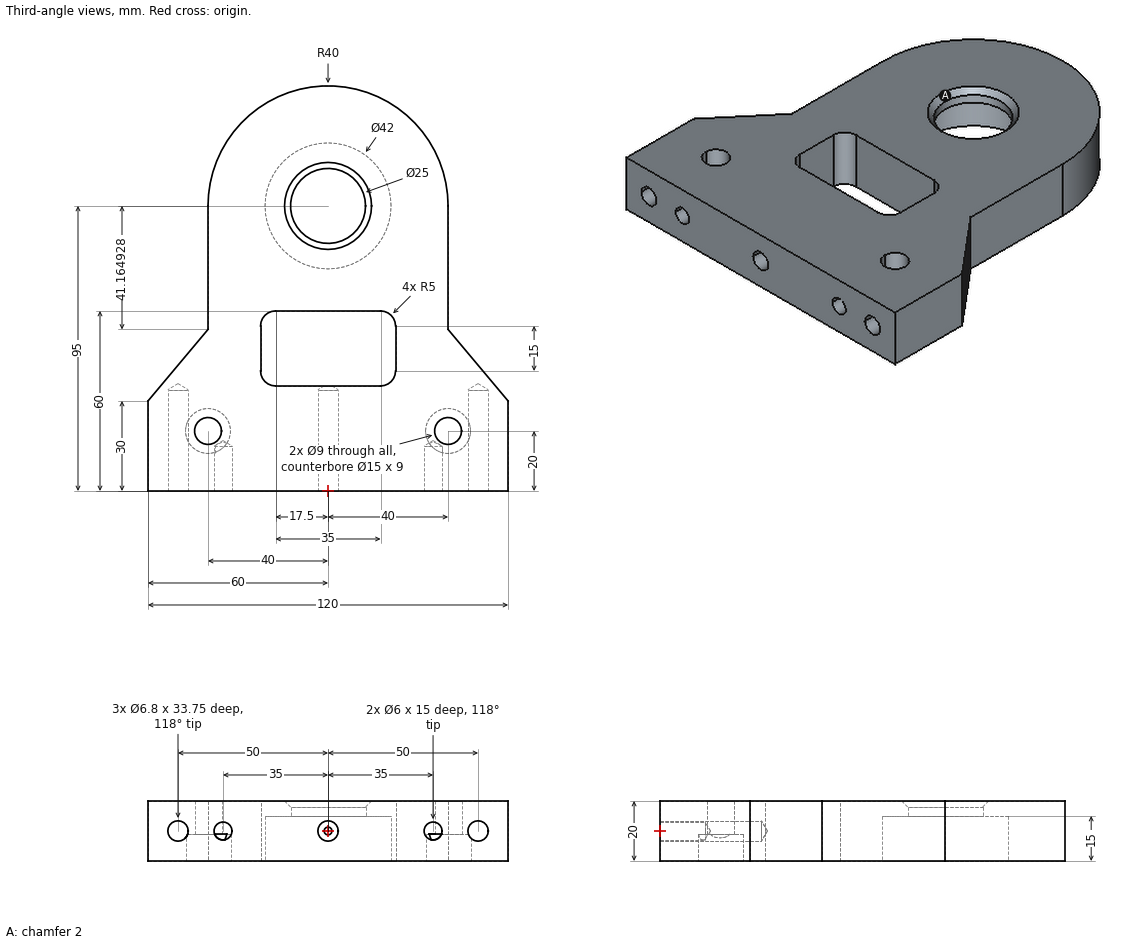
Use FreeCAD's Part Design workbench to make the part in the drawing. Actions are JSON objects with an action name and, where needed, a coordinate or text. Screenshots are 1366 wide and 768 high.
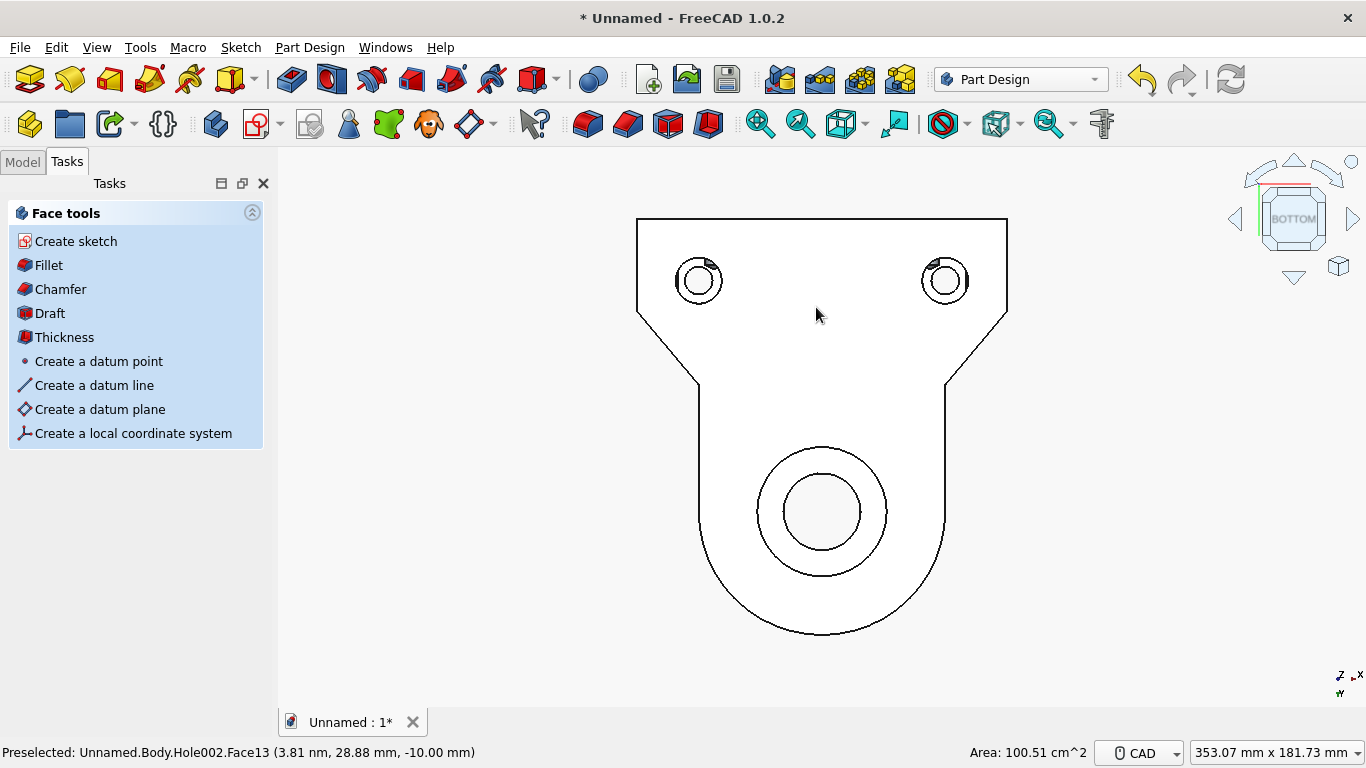
{"action": "left_click", "coordinate": [256, 124]}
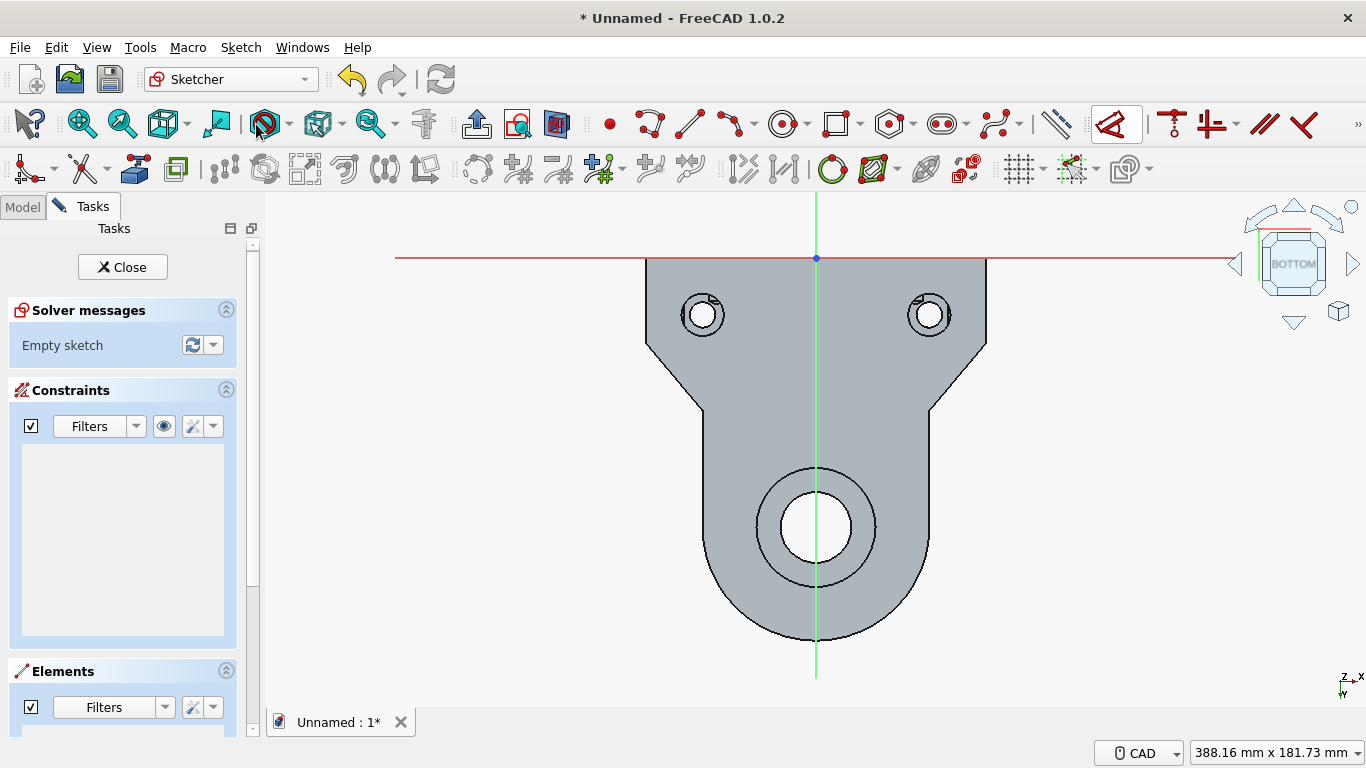
{"action": "scroll", "coordinate": [899, 220], "scroll_direction": "up", "scroll_amount": 3}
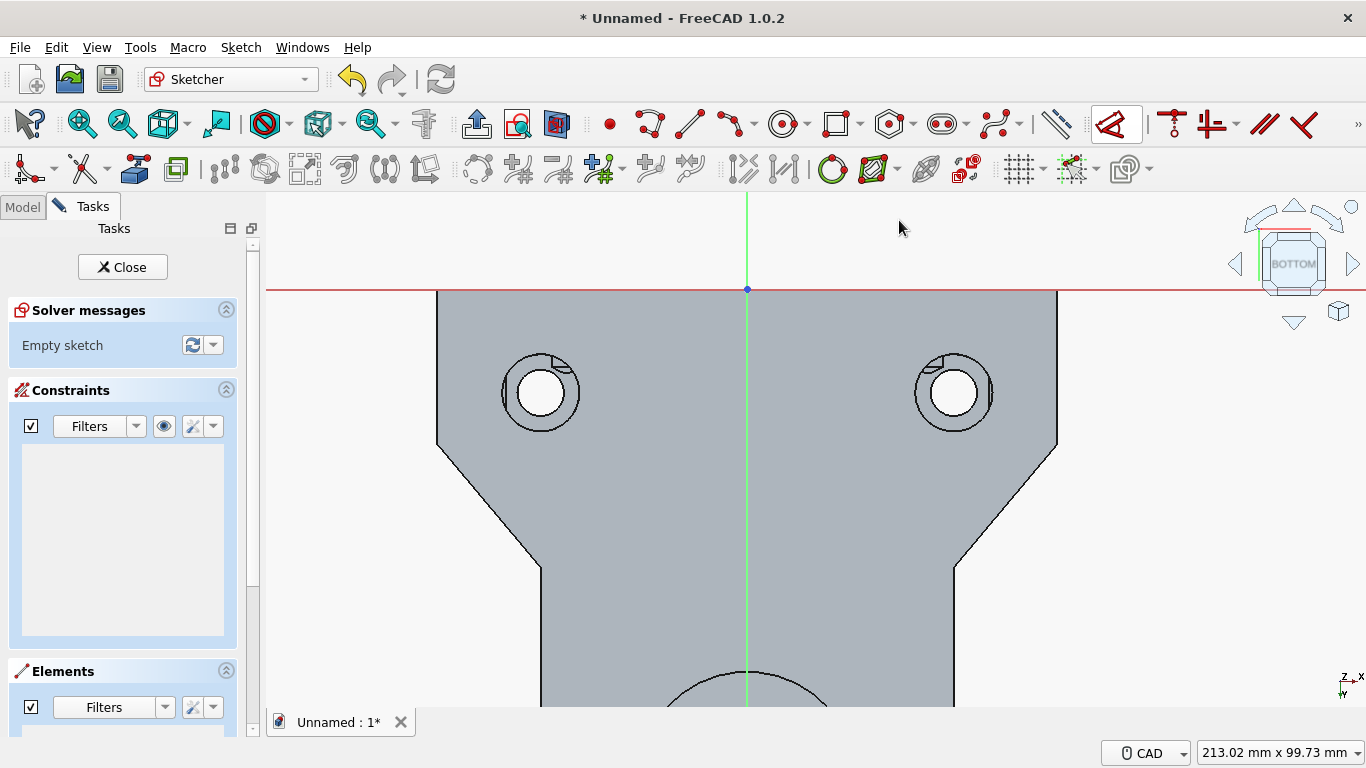
{"action": "key", "text": "g l"}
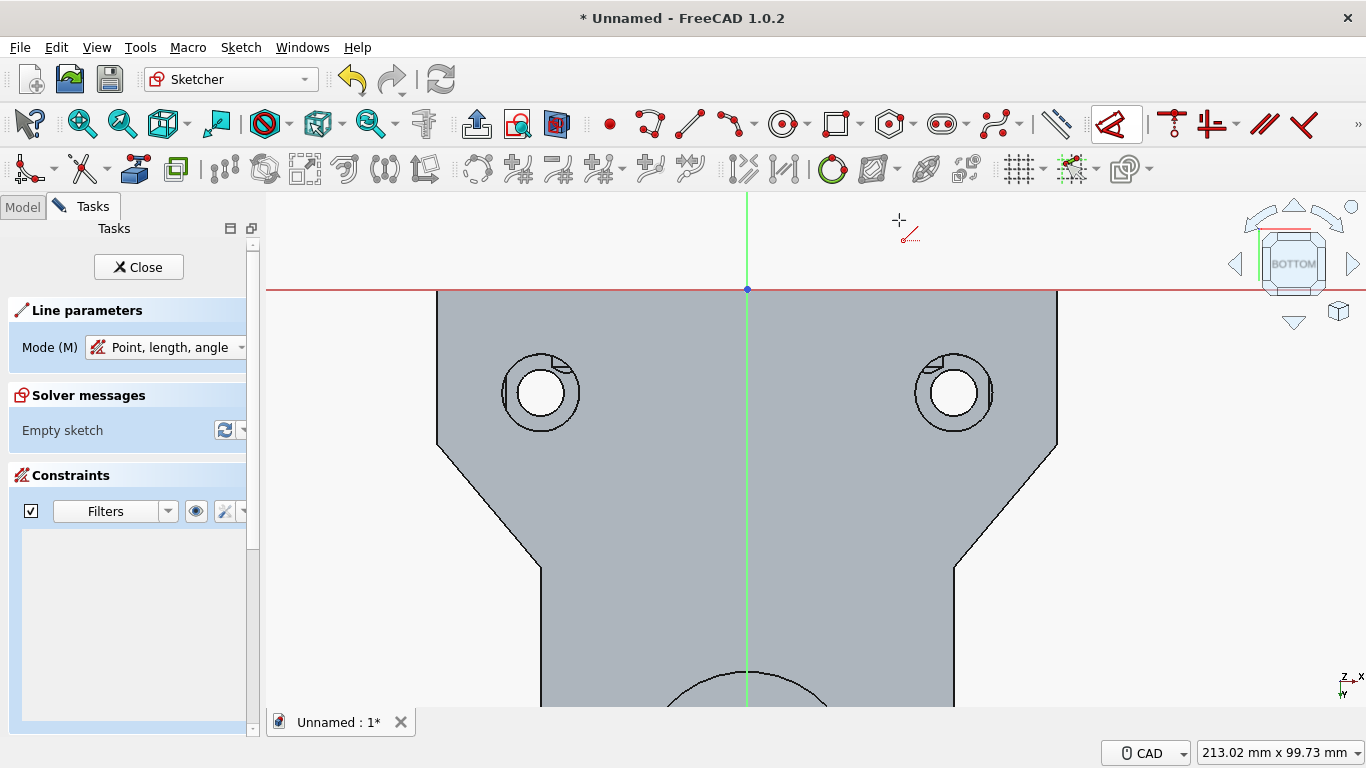
{"action": "left_click", "coordinate": [657, 599]}
{"action": "left_click", "coordinate": [838, 599]}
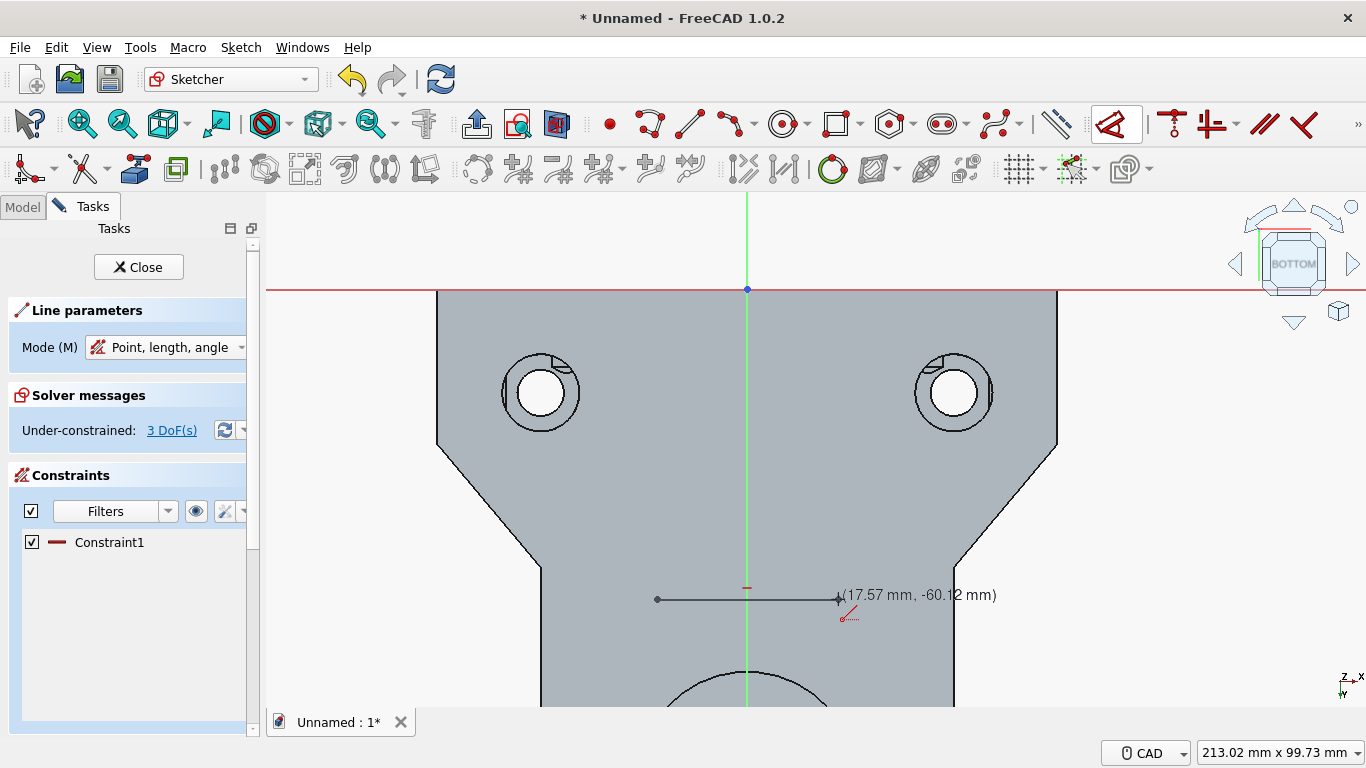
{"action": "left_click", "coordinate": [863, 574]}
{"action": "left_click", "coordinate": [863, 496]}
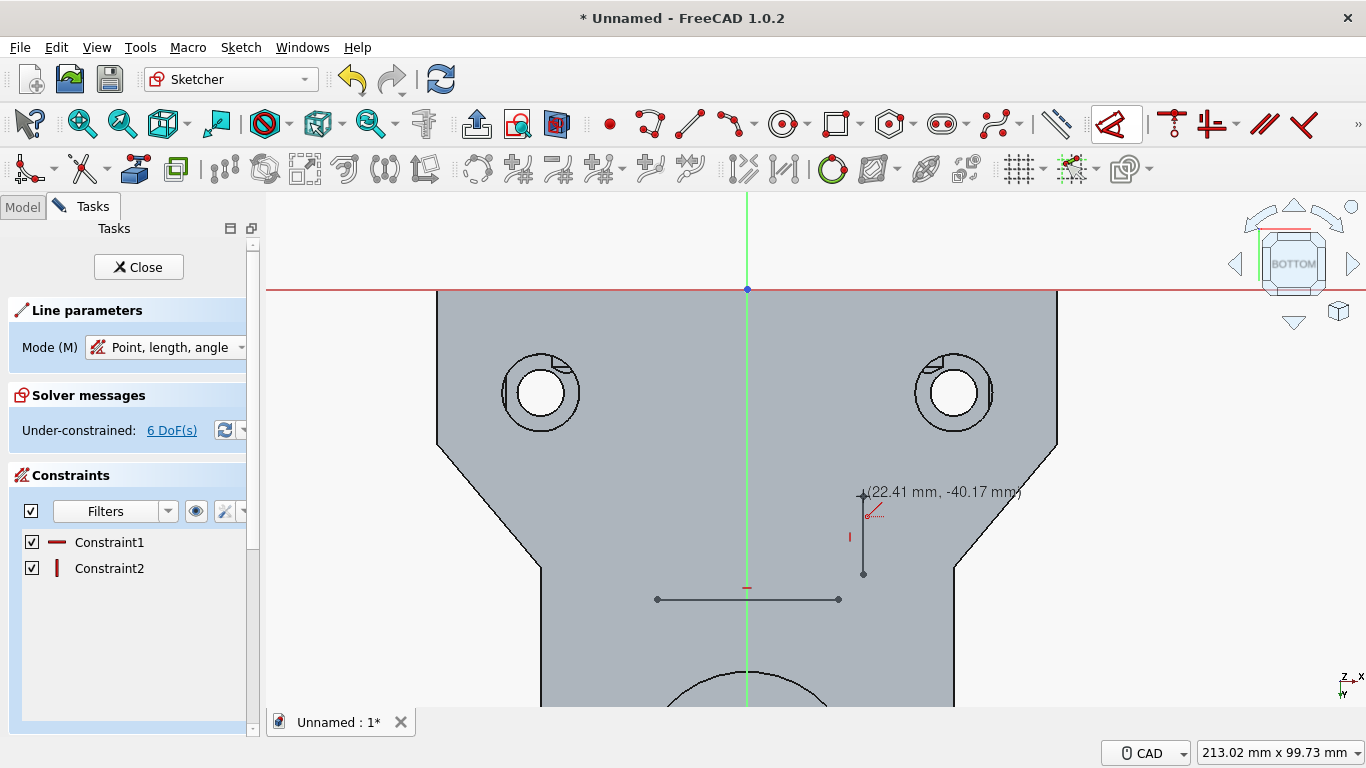
{"action": "left_click", "coordinate": [838, 470]}
{"action": "left_click", "coordinate": [657, 470]}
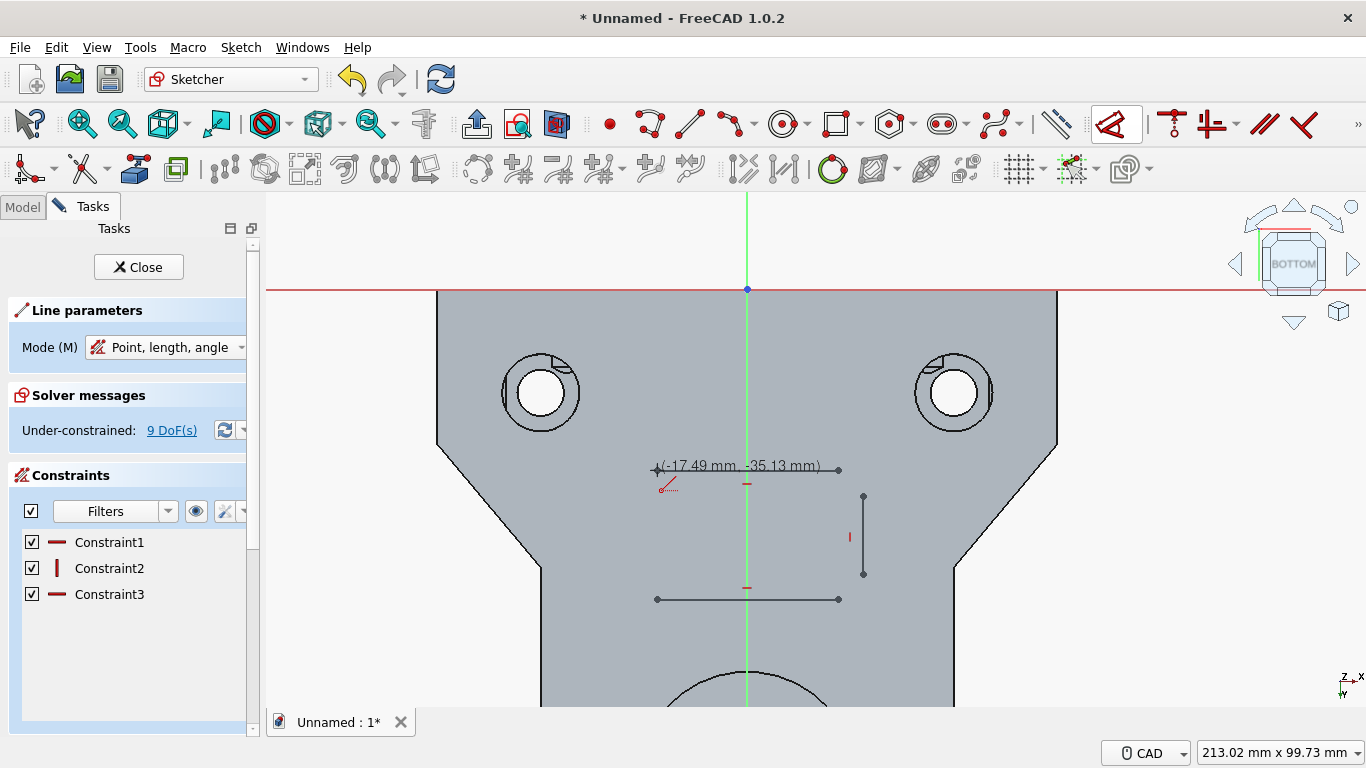
{"action": "left_click", "coordinate": [631, 496]}
{"action": "left_click", "coordinate": [631, 574]}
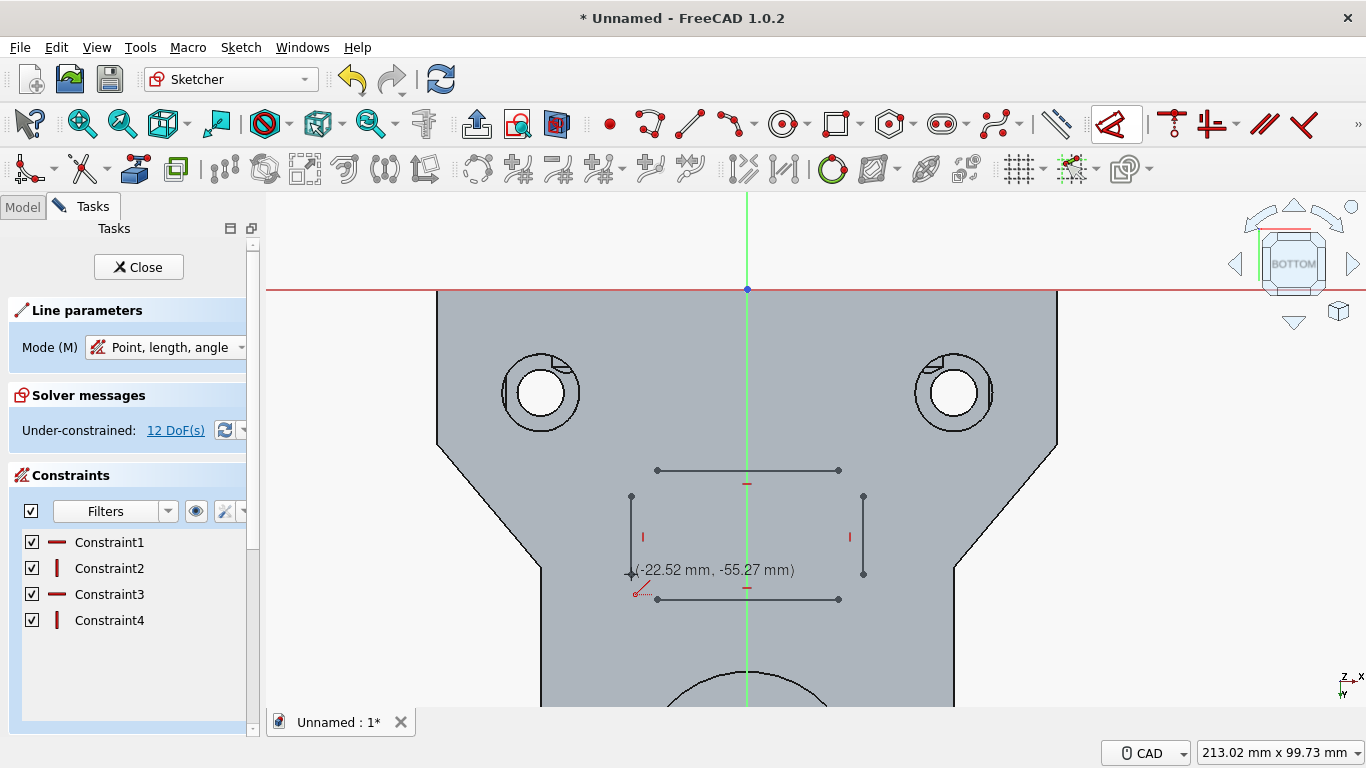
{"action": "left_click", "coordinate": [730, 124]}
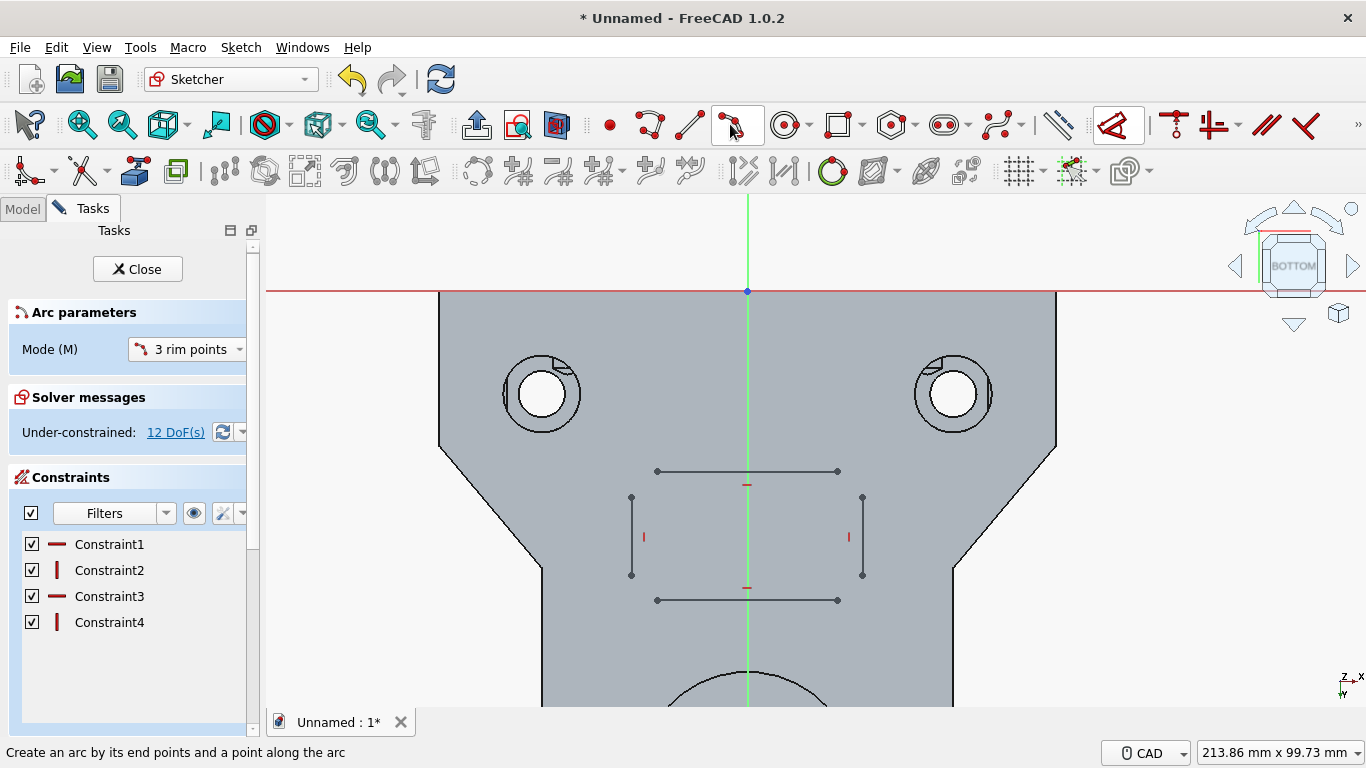
{"action": "left_click", "coordinate": [838, 600]}
{"action": "left_click", "coordinate": [863, 576]}